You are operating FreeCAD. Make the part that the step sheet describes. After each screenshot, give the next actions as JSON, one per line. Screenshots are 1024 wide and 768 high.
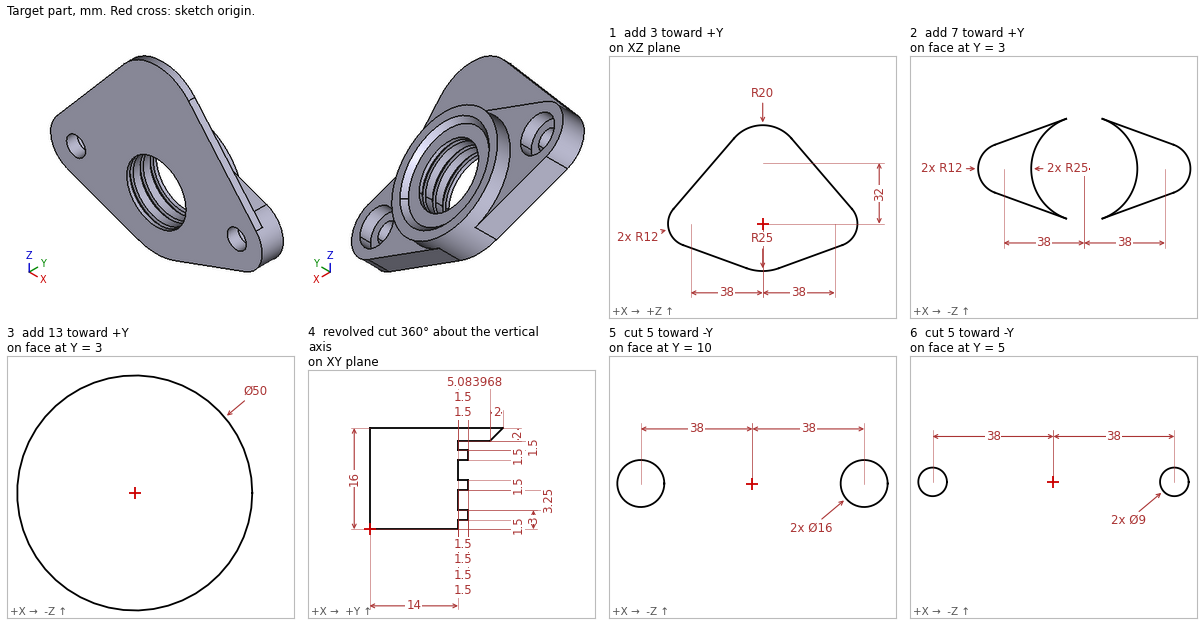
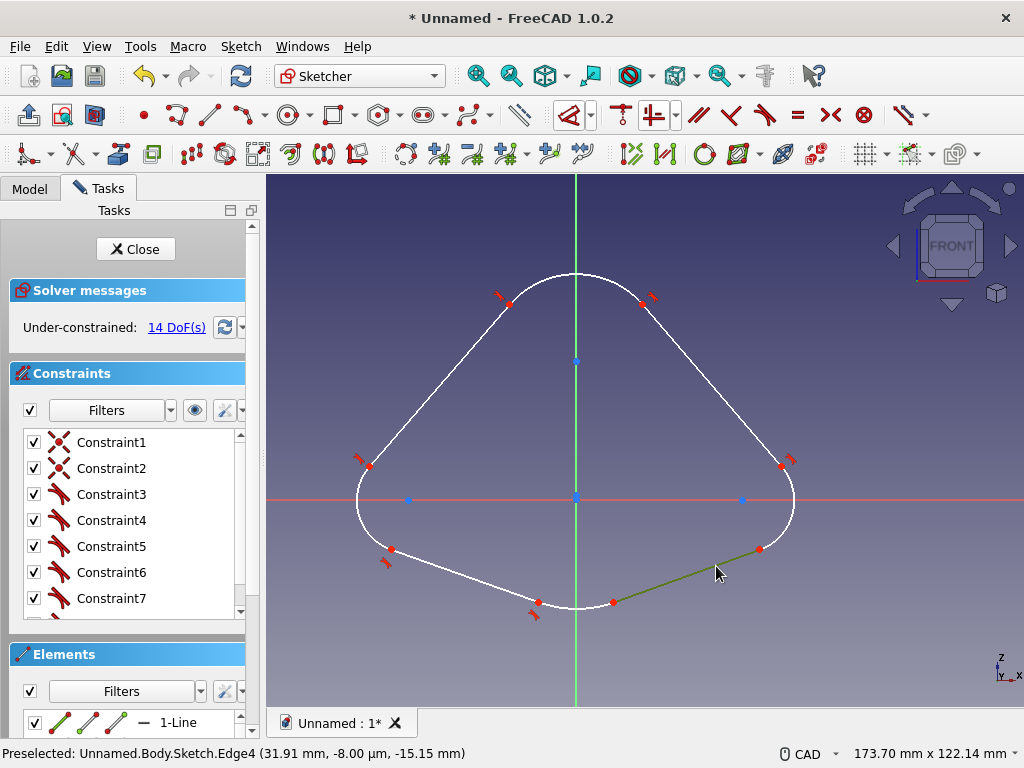
{"action": "left_click", "coordinate": [784, 532]}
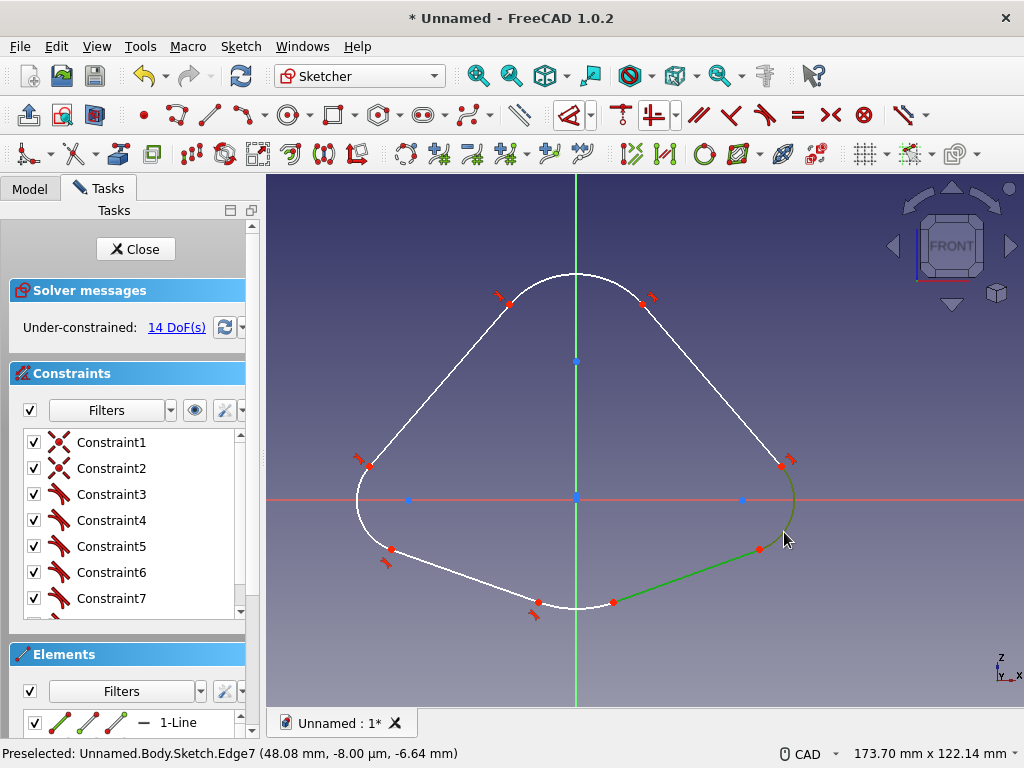
{"action": "left_click", "coordinate": [765, 116]}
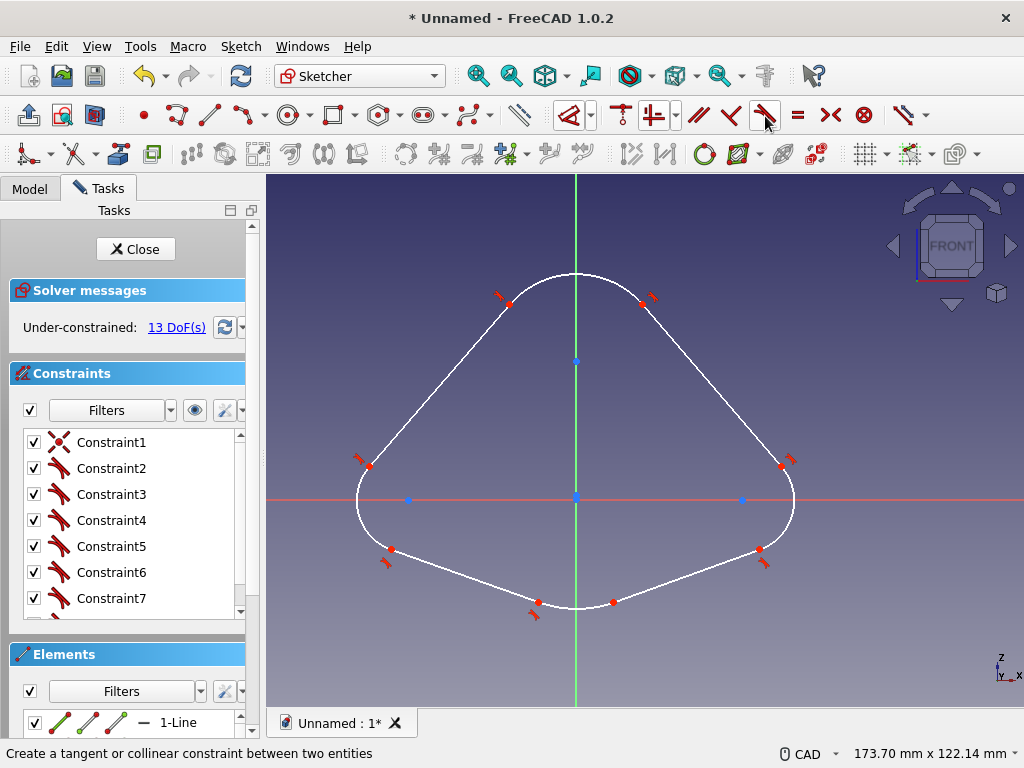
{"action": "left_click", "coordinate": [716, 566]}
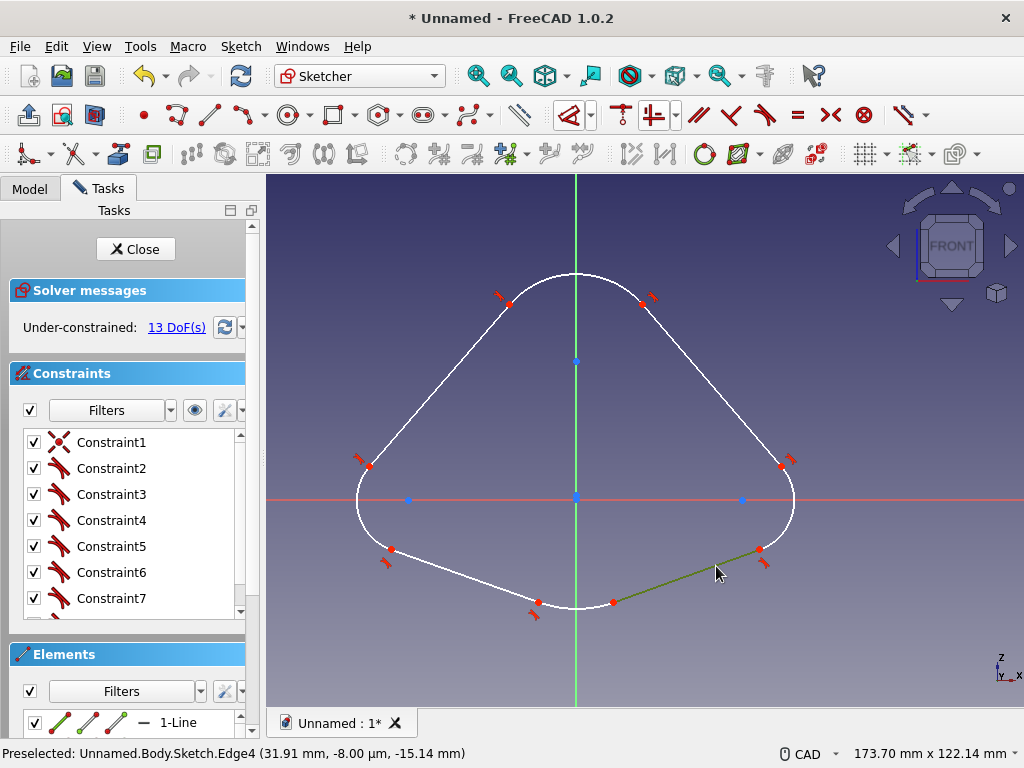
{"action": "left_click", "coordinate": [561, 608]}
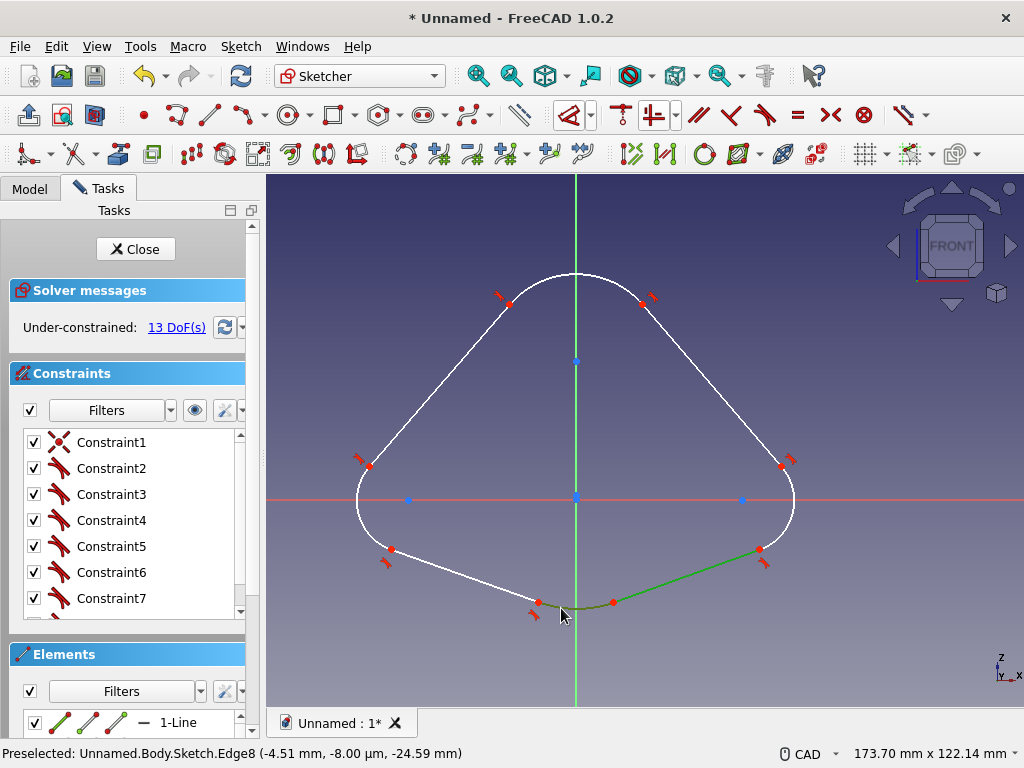
{"action": "left_click", "coordinate": [765, 116]}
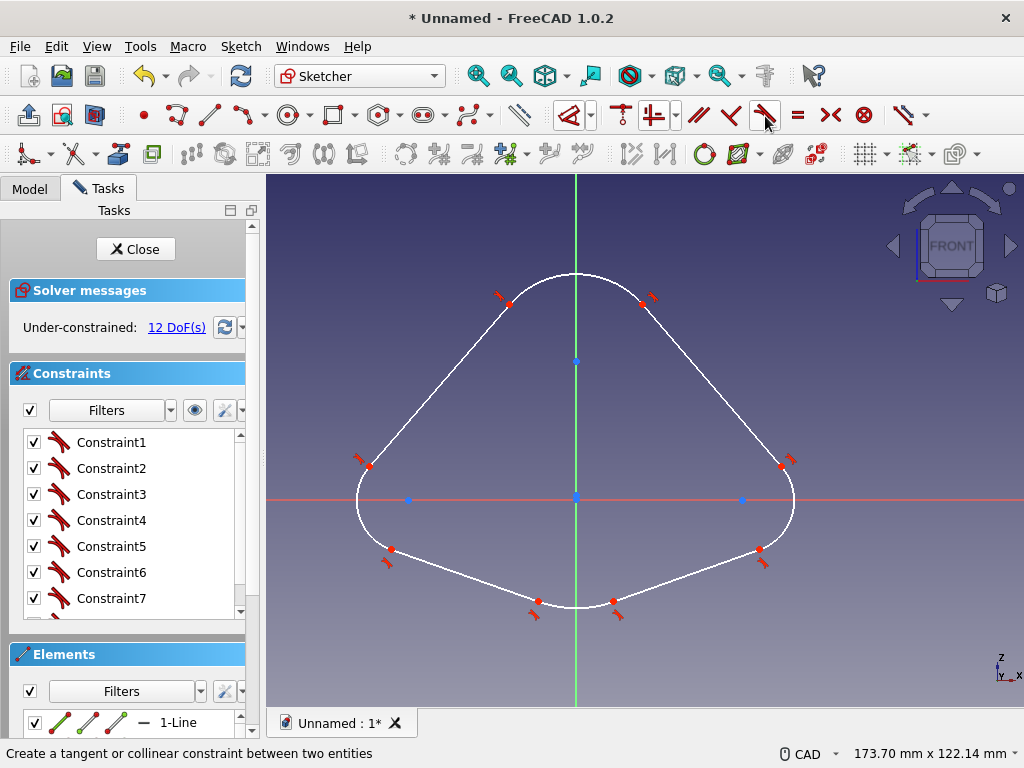
{"action": "left_click_drag", "start_coordinate": [566, 486], "coordinate": [586, 510]}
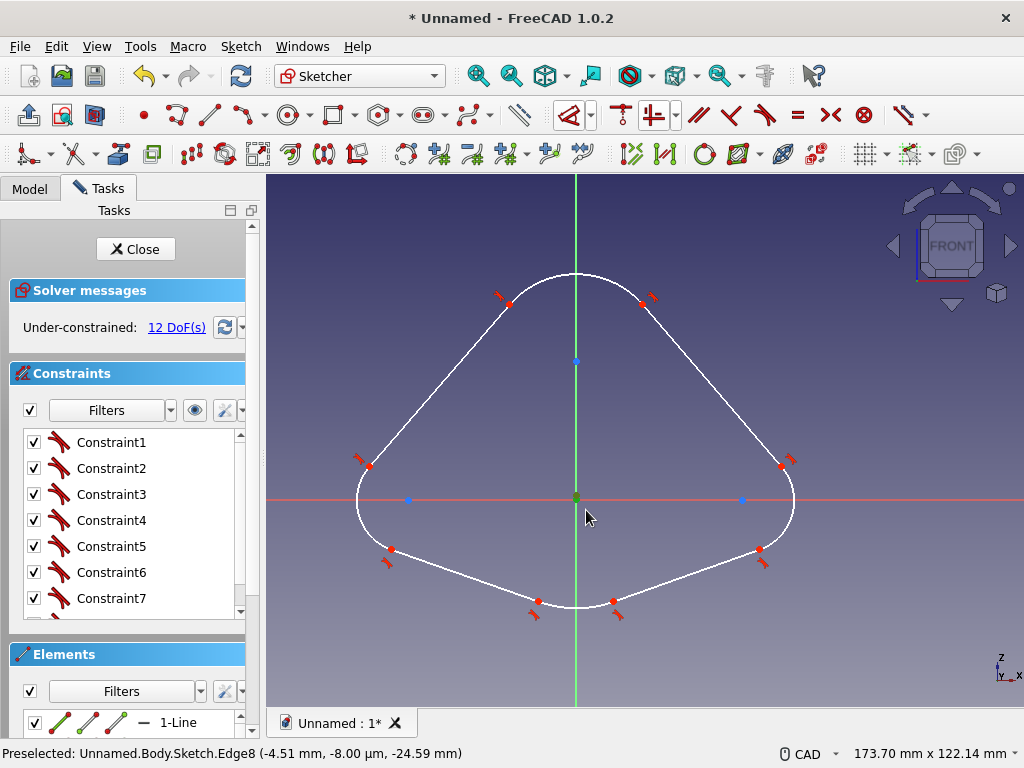
{"action": "left_click", "coordinate": [621, 116]}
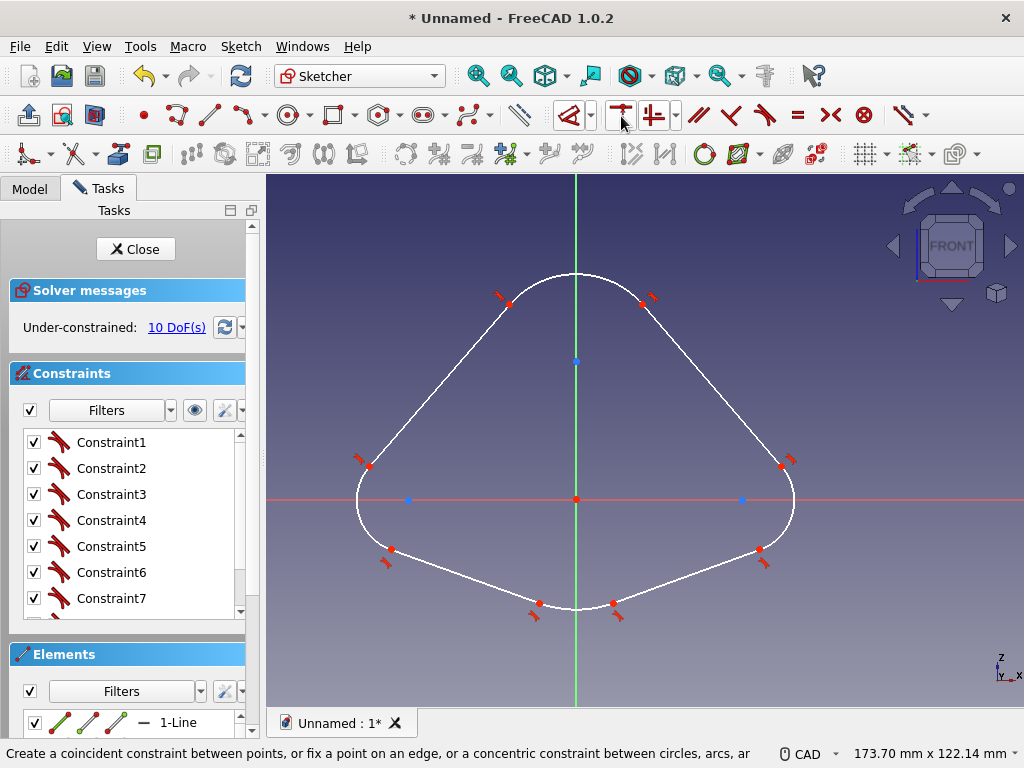
{"action": "left_click", "coordinate": [367, 532]}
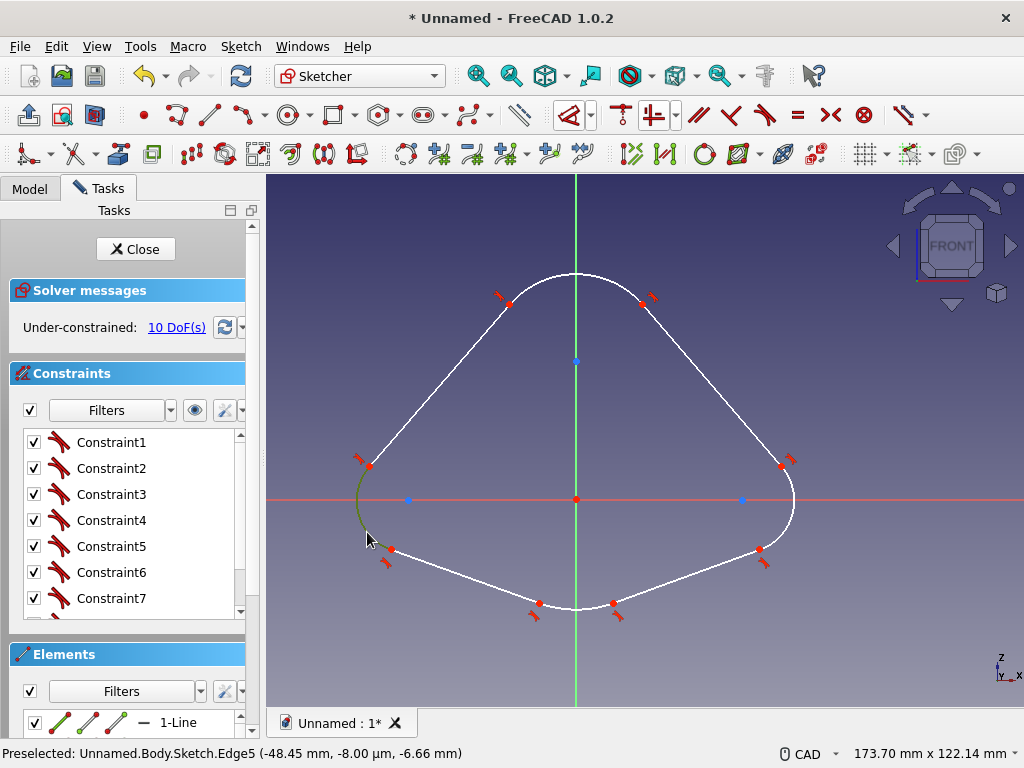
{"action": "left_click", "coordinate": [784, 532]}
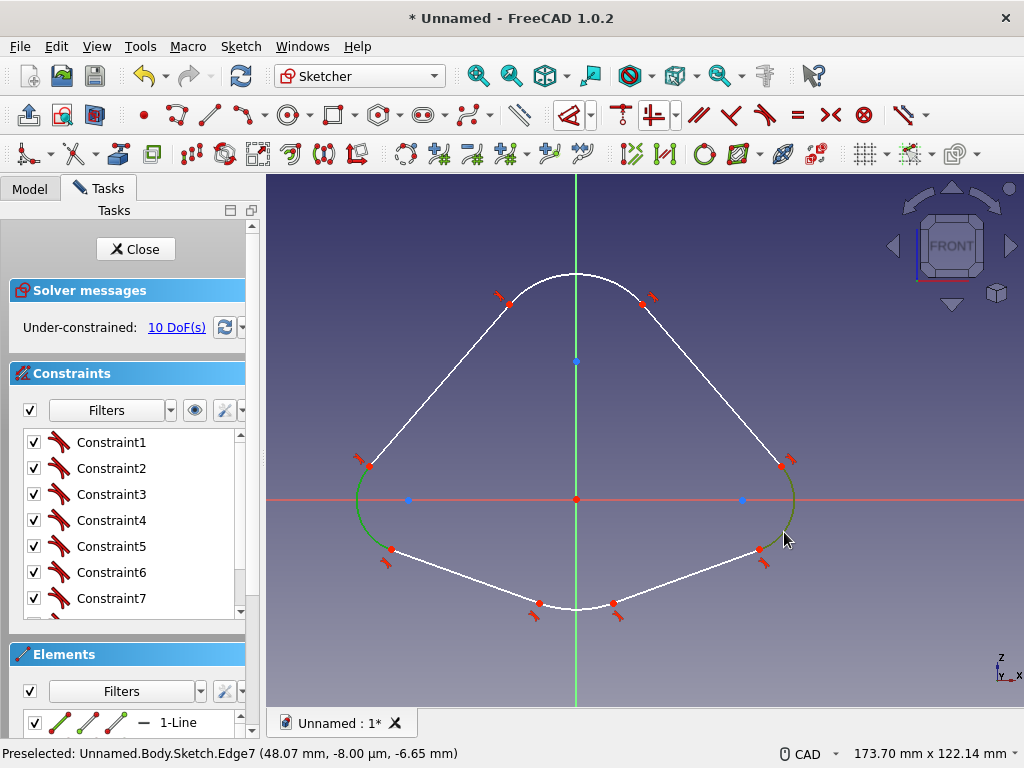
{"action": "left_click", "coordinate": [798, 116]}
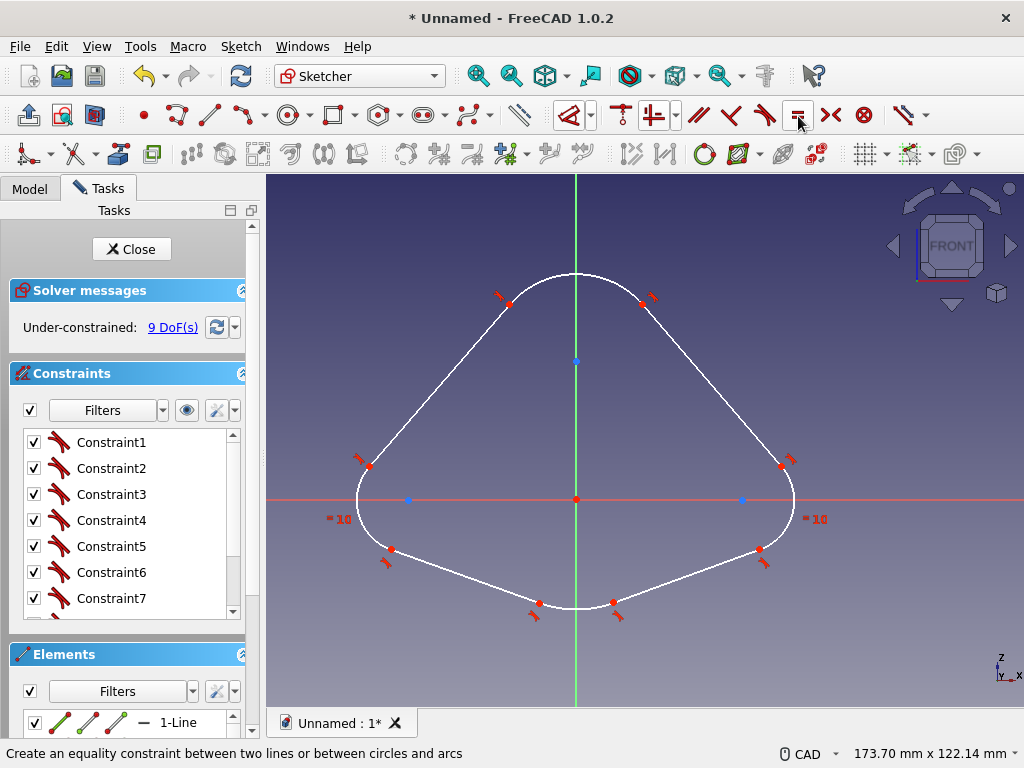
{"action": "left_click", "coordinate": [409, 501]}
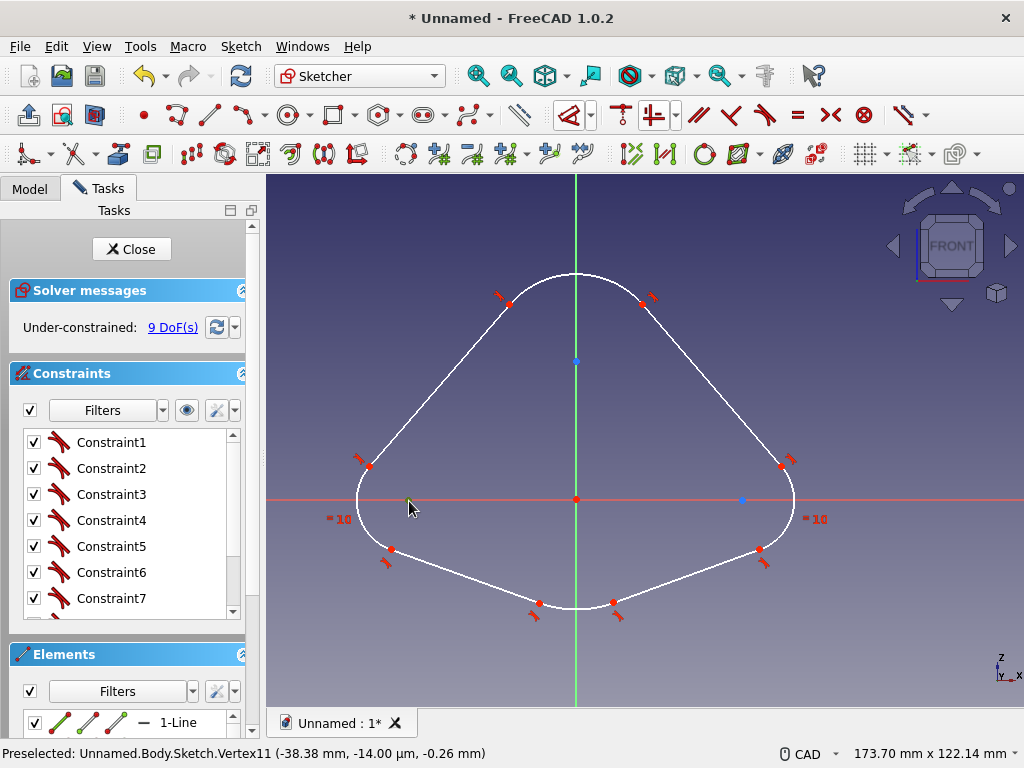
{"action": "left_click", "coordinate": [415, 500]}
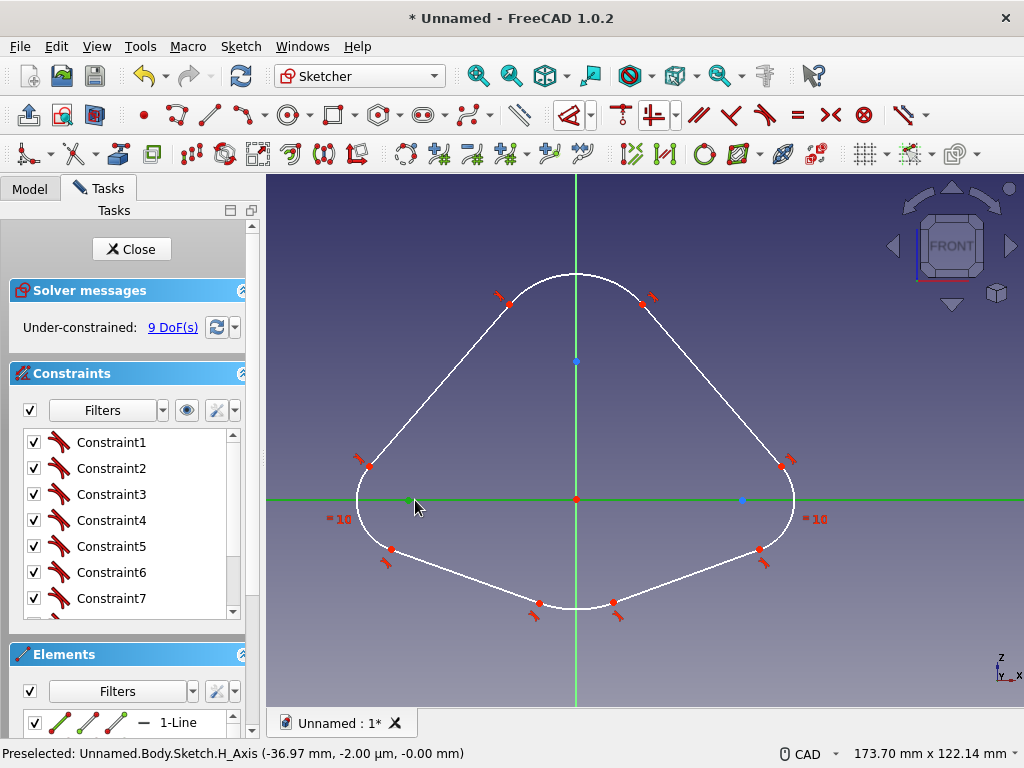
{"action": "left_click", "coordinate": [621, 116]}